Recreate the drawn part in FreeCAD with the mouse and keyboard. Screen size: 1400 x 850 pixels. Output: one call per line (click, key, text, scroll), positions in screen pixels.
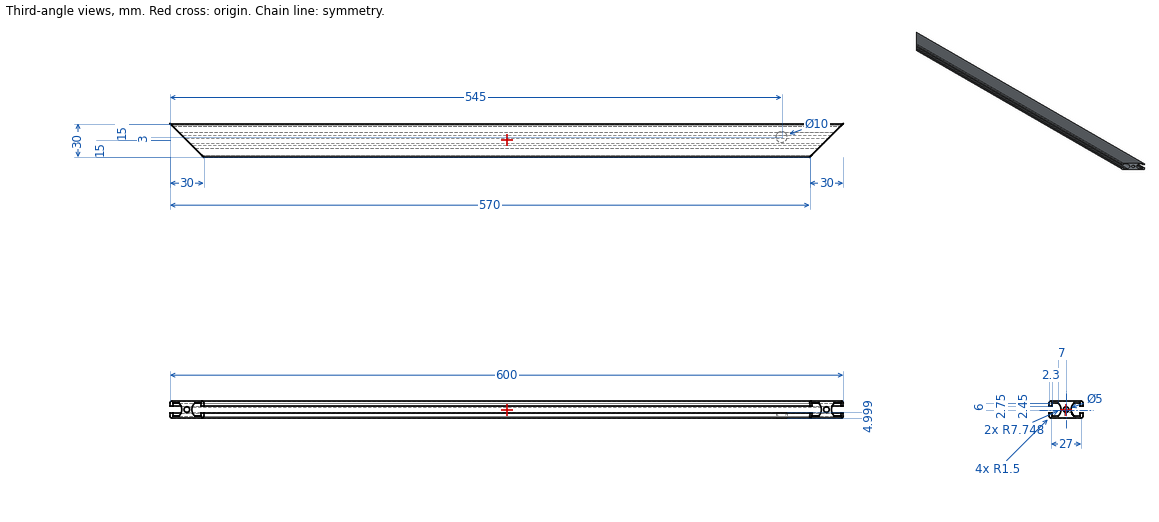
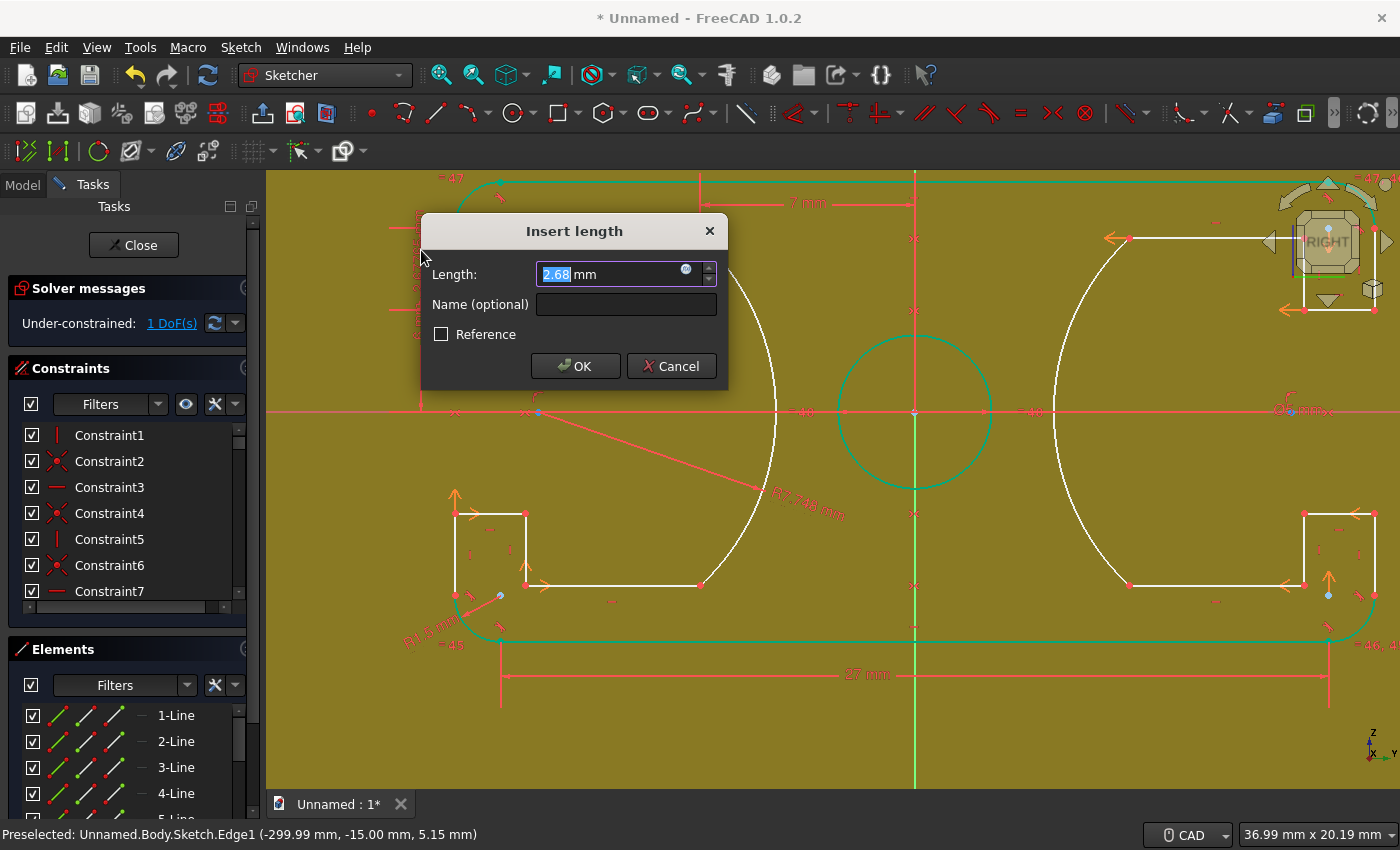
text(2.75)
key(Return)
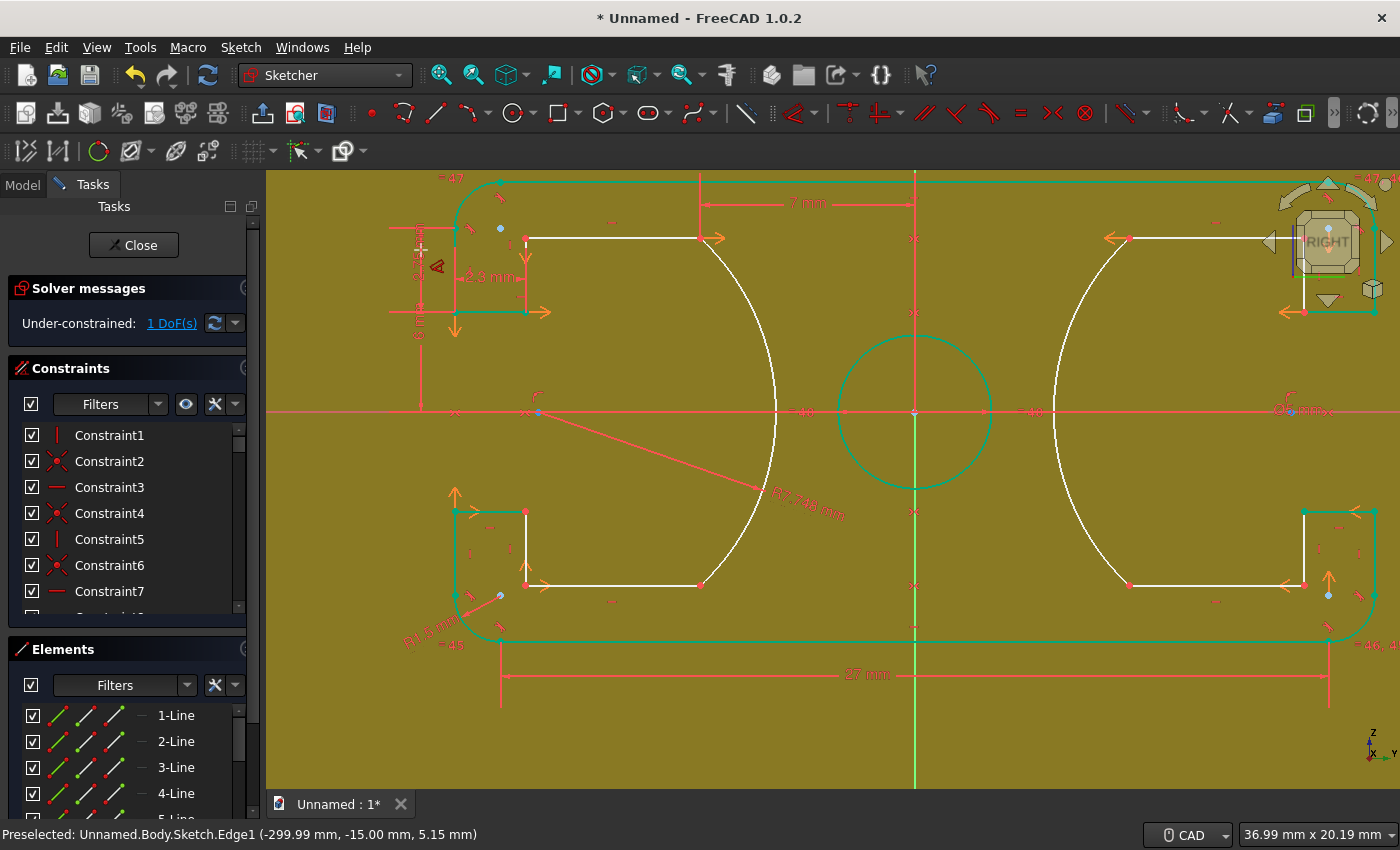
click(526, 290)
click(492, 249)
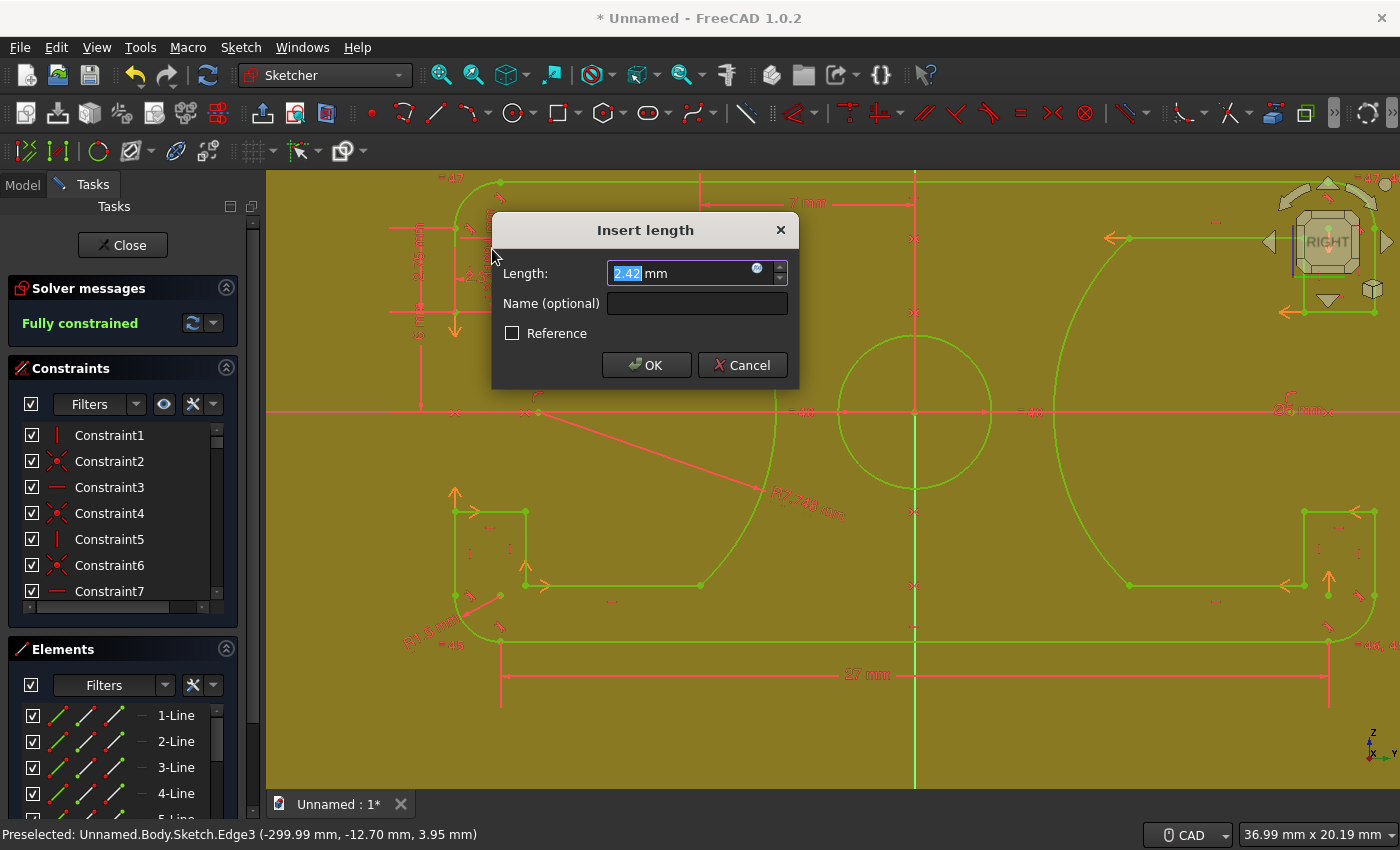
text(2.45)
key(Return)
key(Escape)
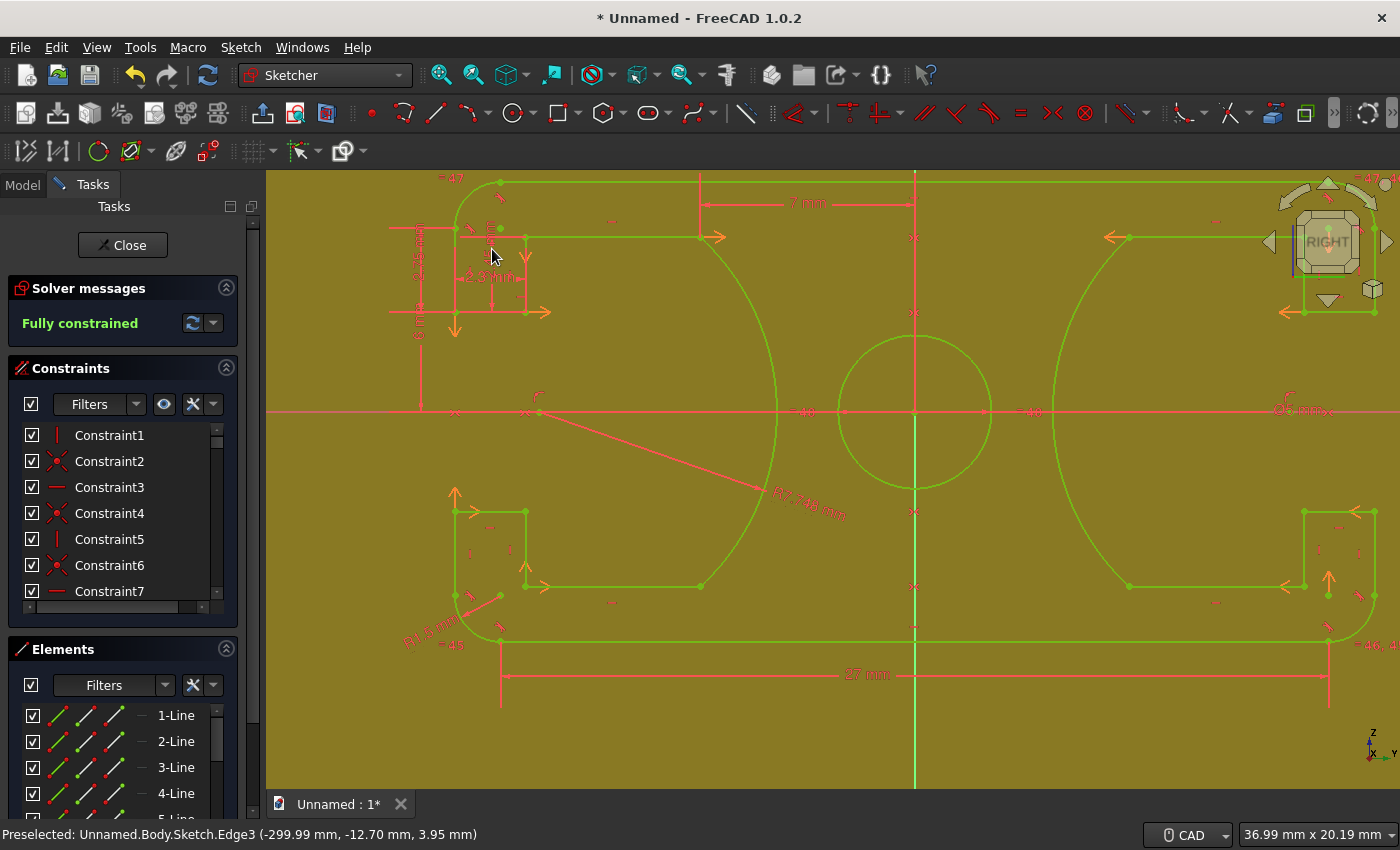
click(123, 245)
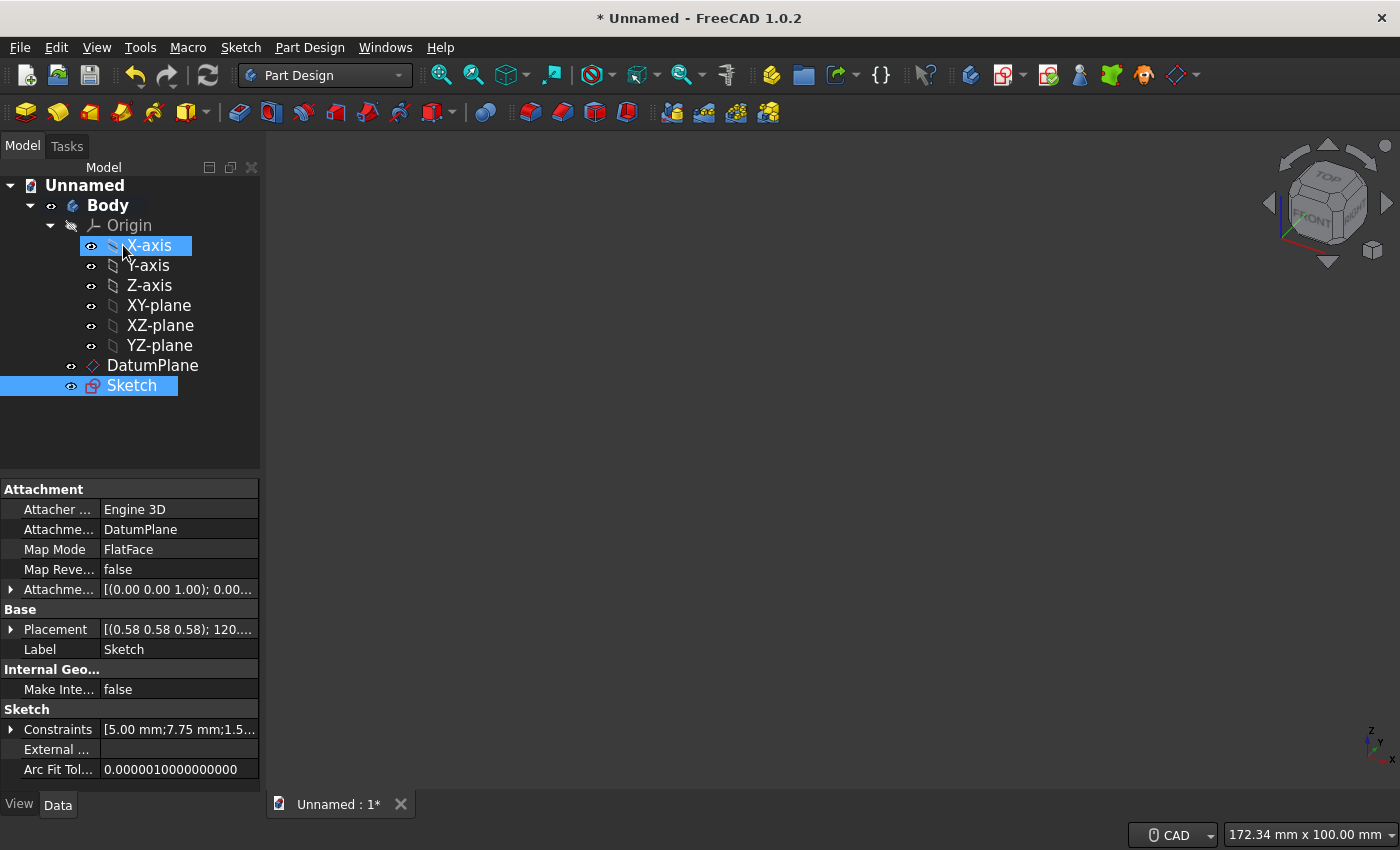
click(26, 112)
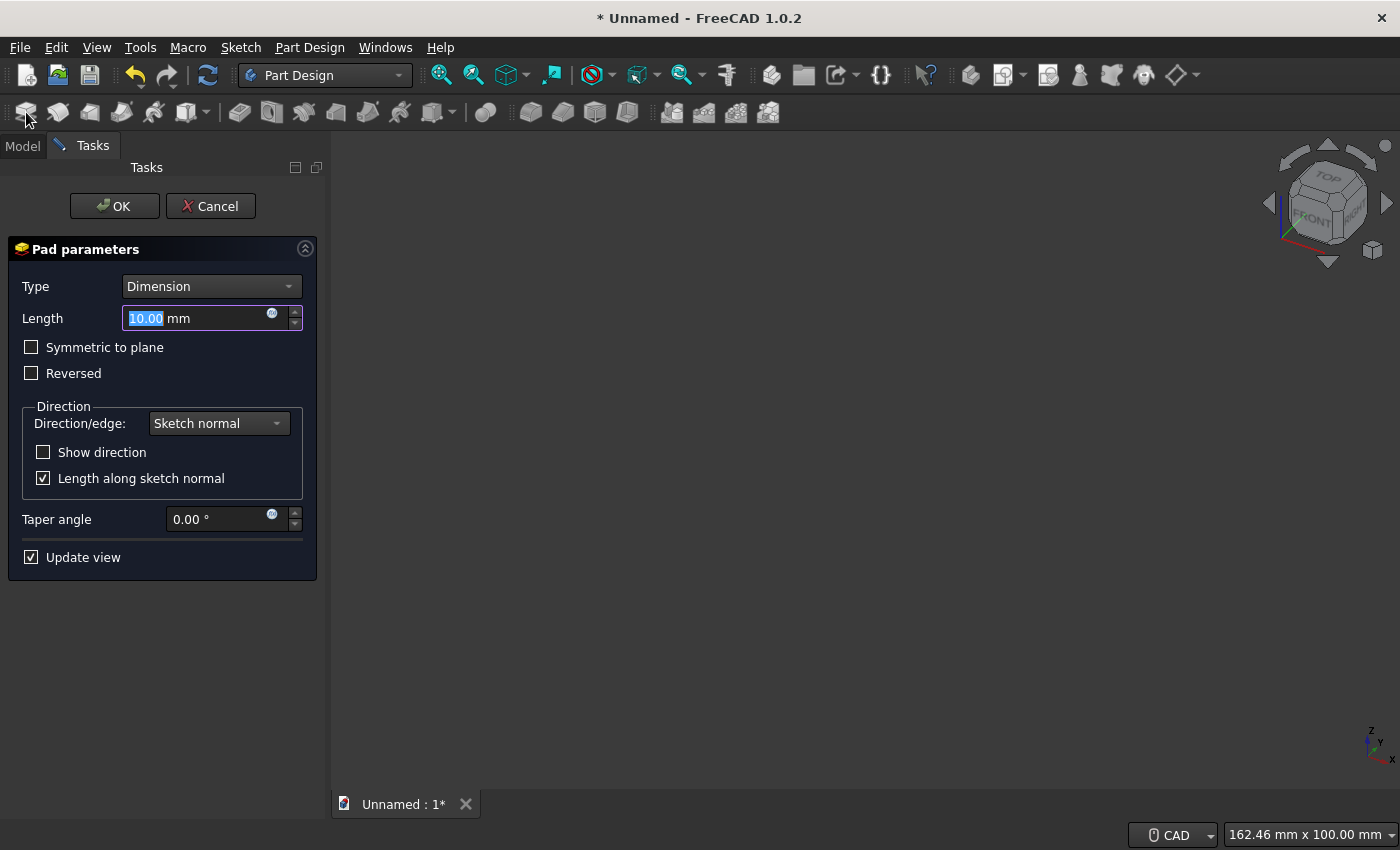
text(600)
key(Tab)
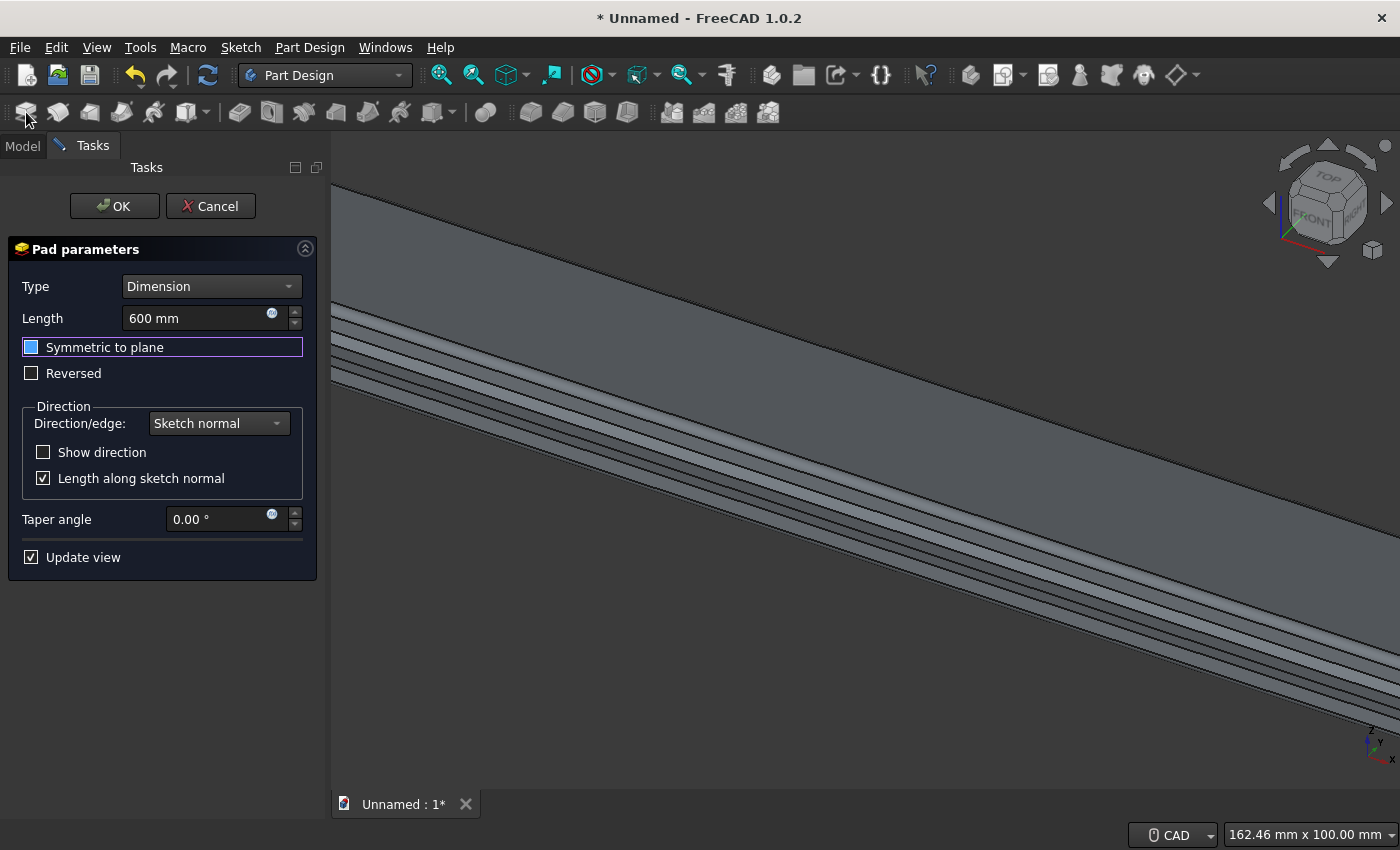
click(115, 206)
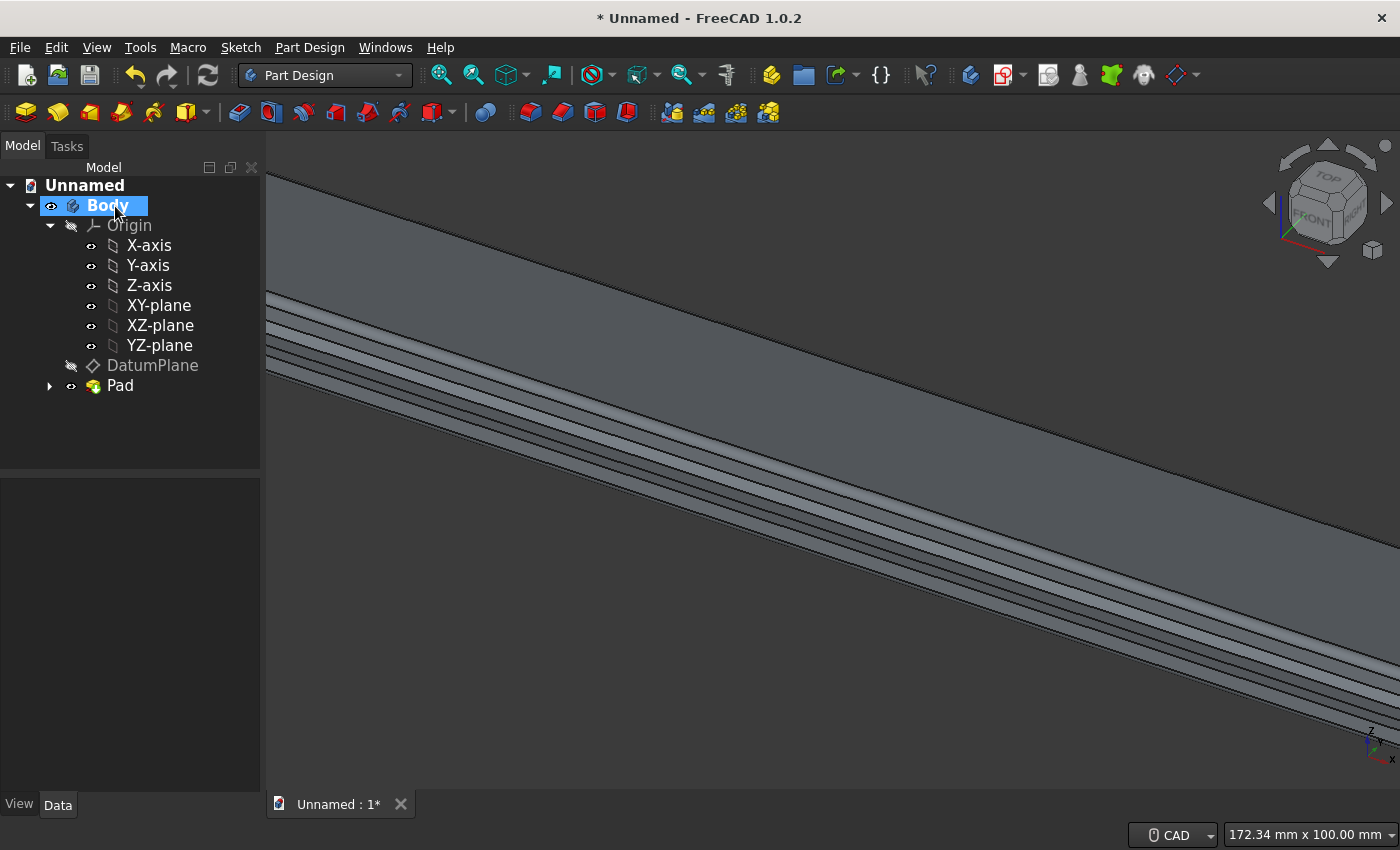
key(v)
key(f)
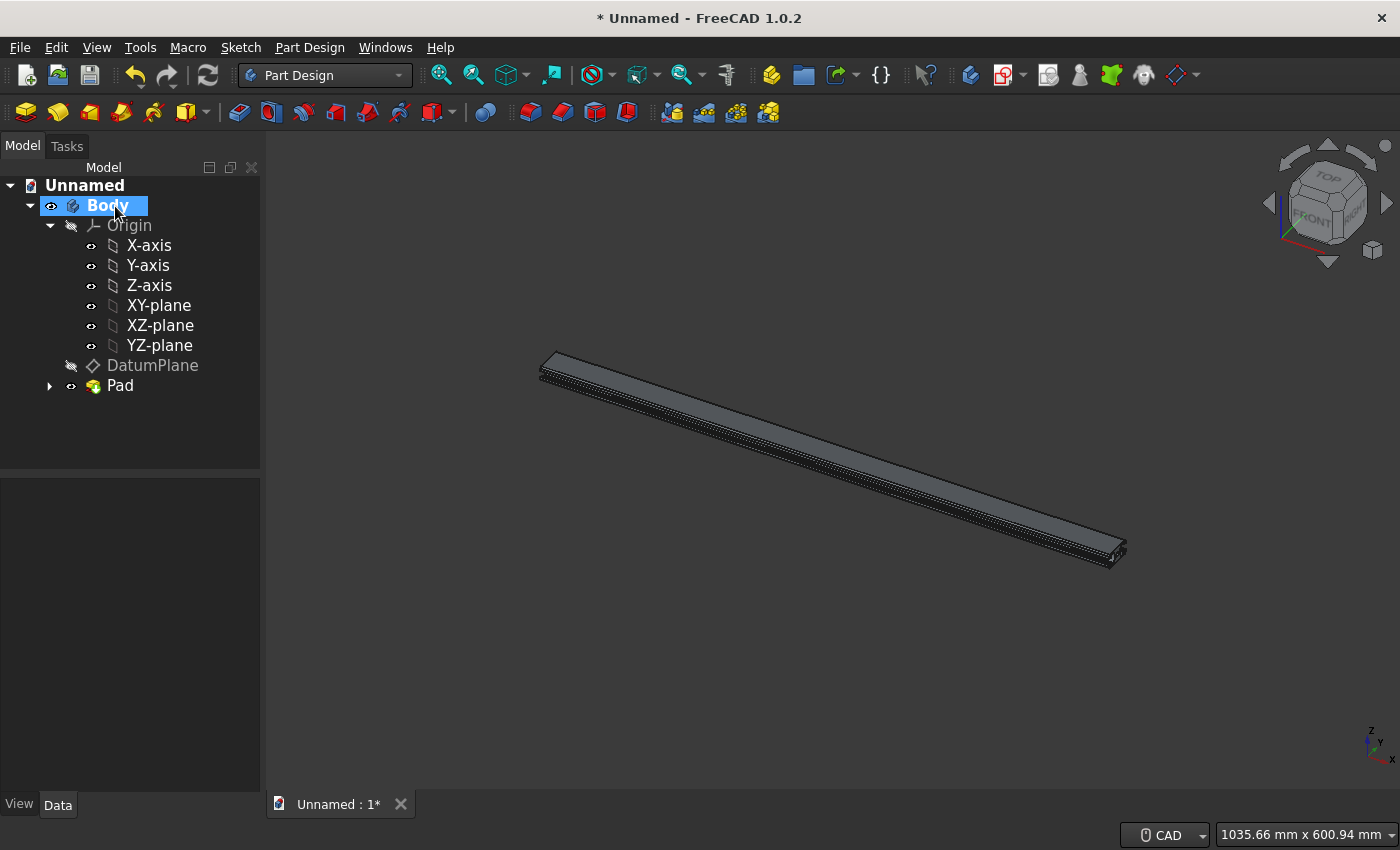
key(0)